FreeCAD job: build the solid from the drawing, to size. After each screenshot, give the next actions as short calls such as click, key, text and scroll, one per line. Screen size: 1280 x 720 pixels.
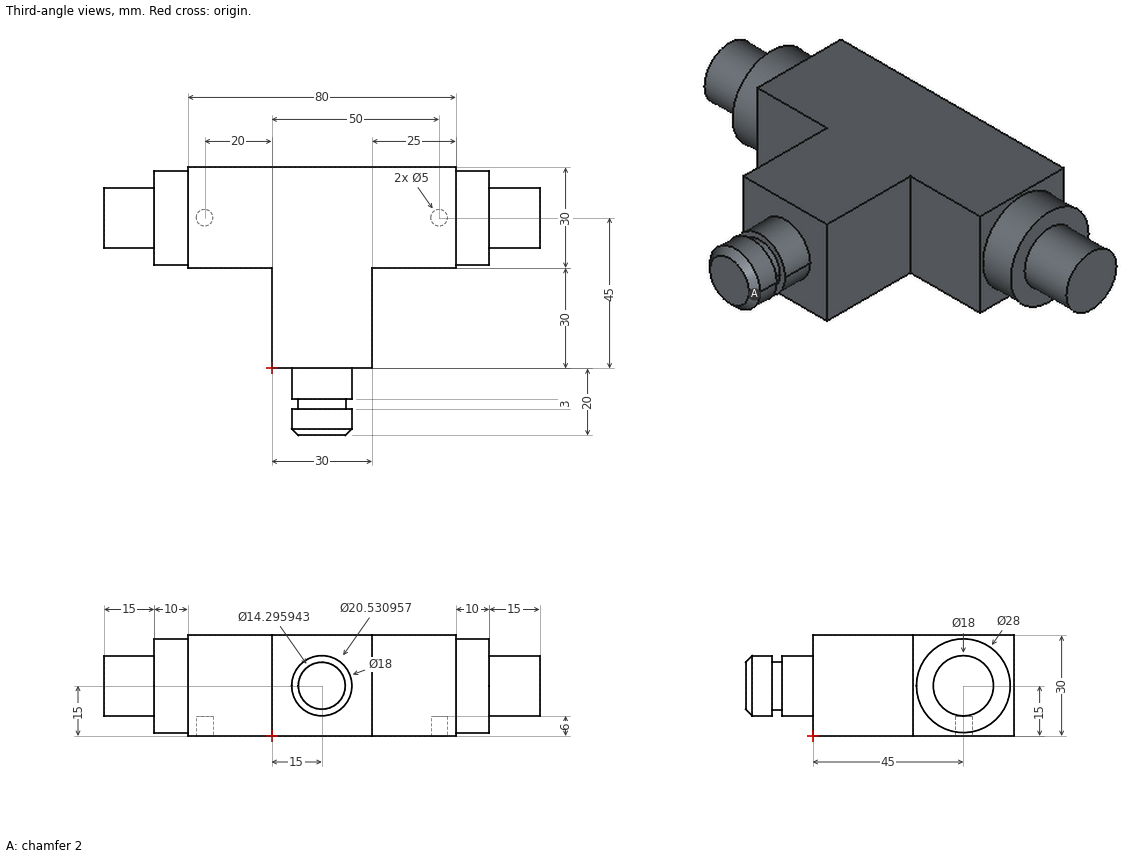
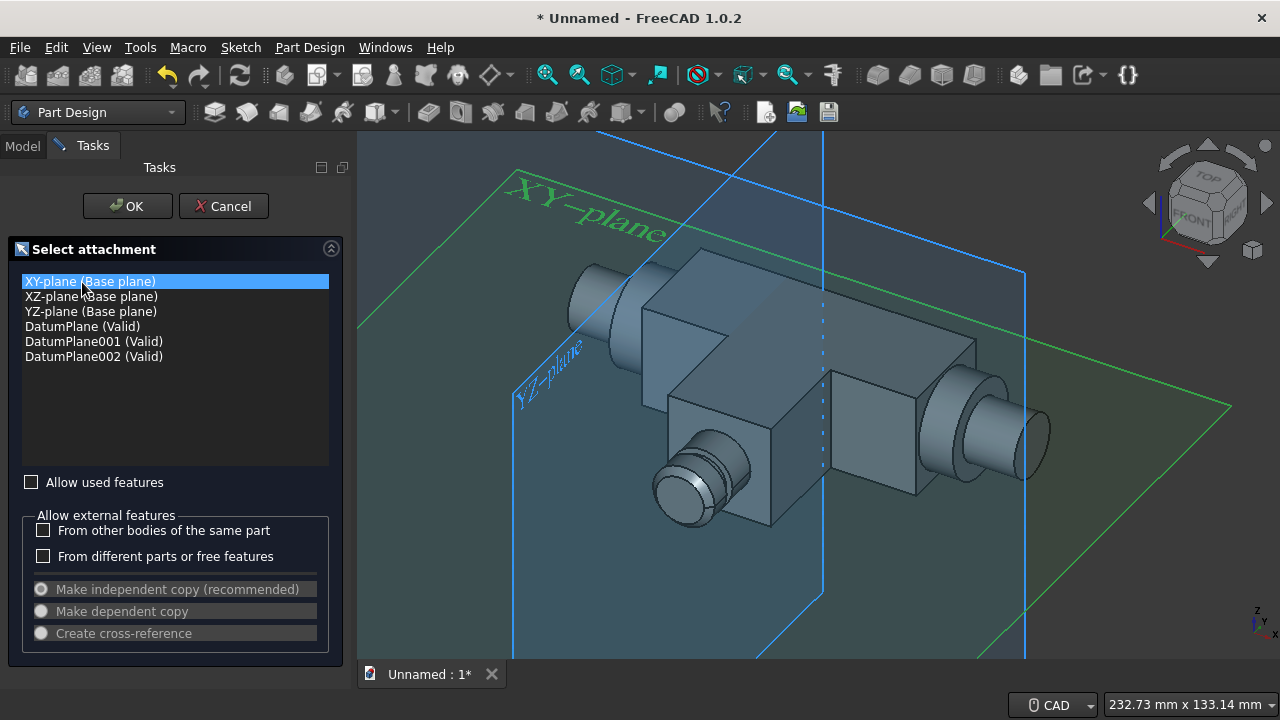
click(128, 206)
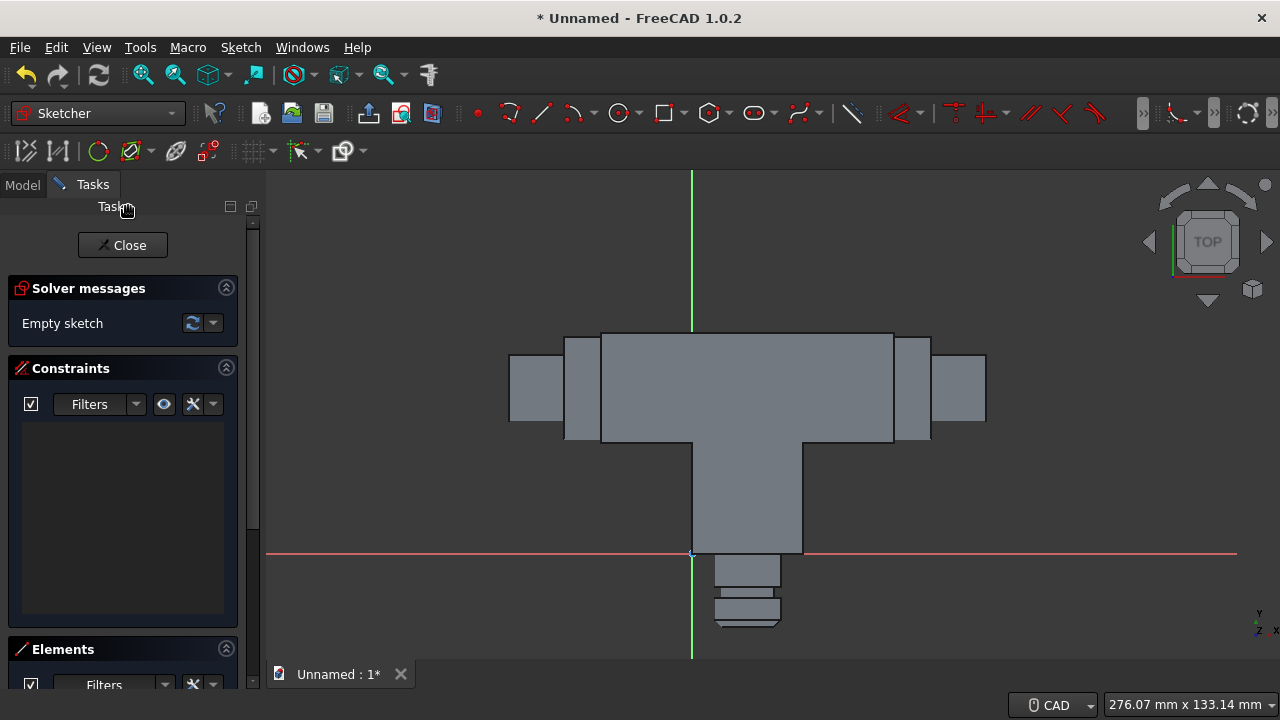
click(434, 114)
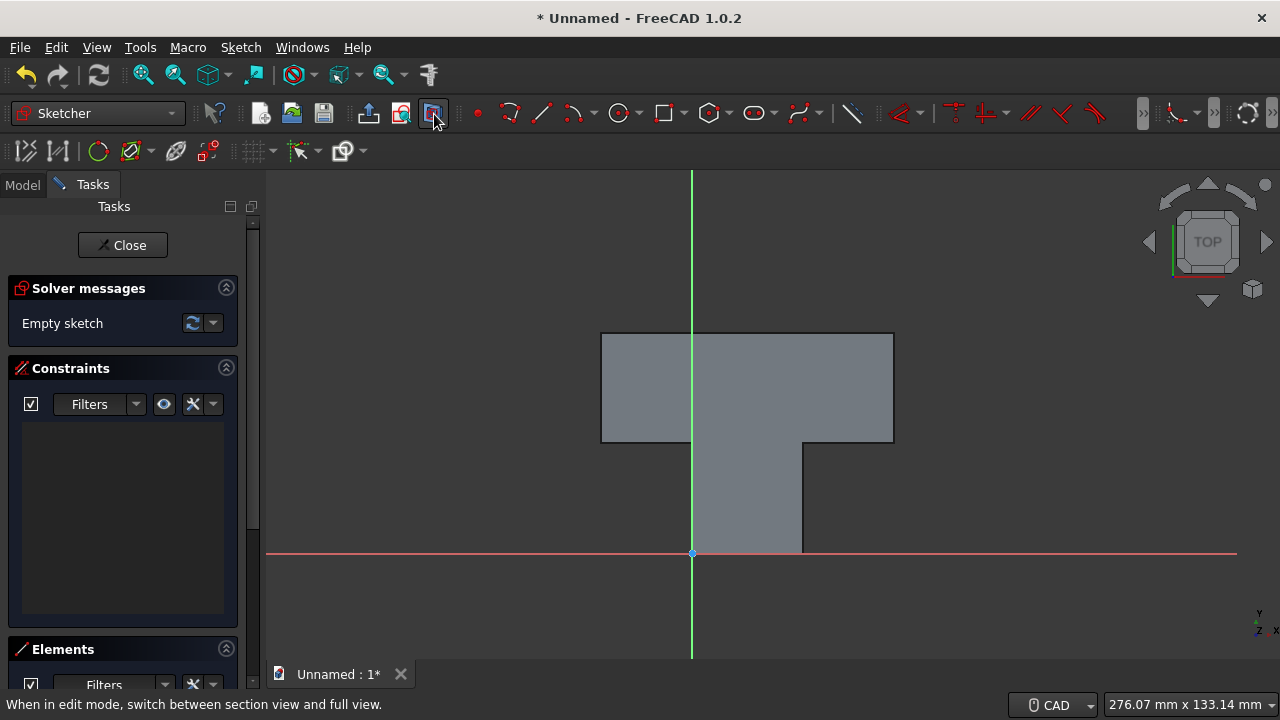
scroll(800, 530, up, 3)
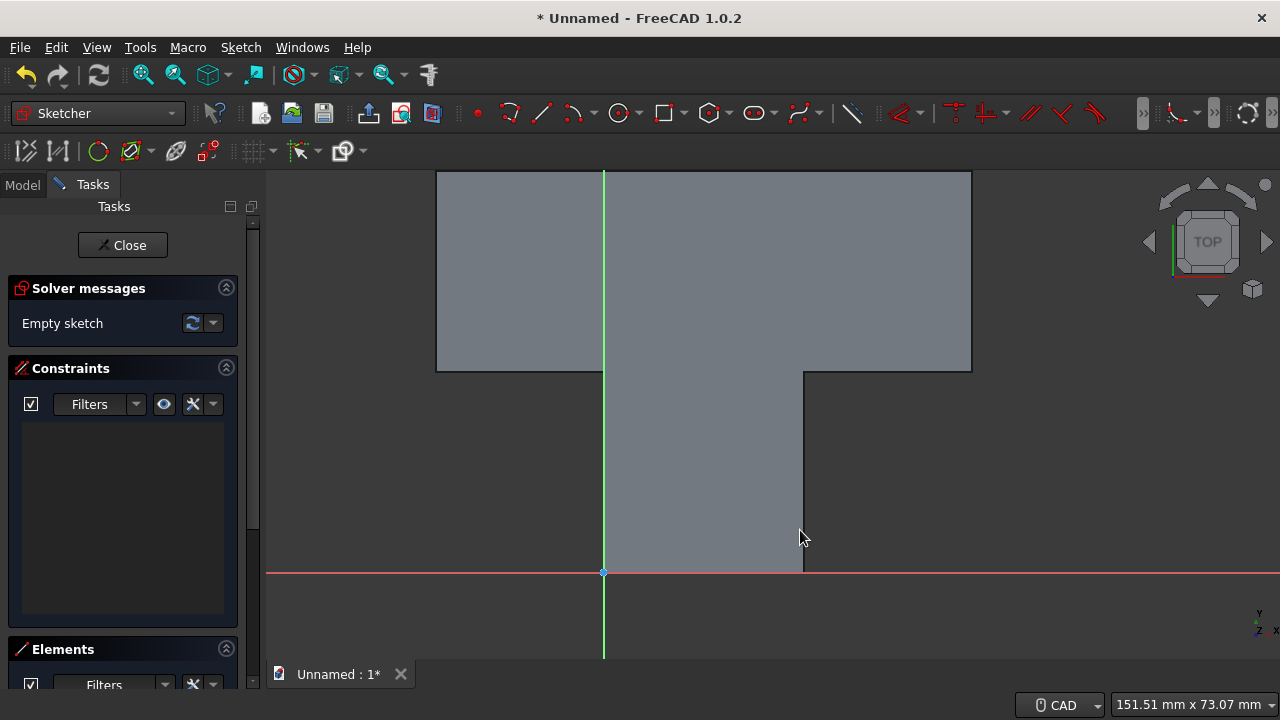
key(g)
key(c)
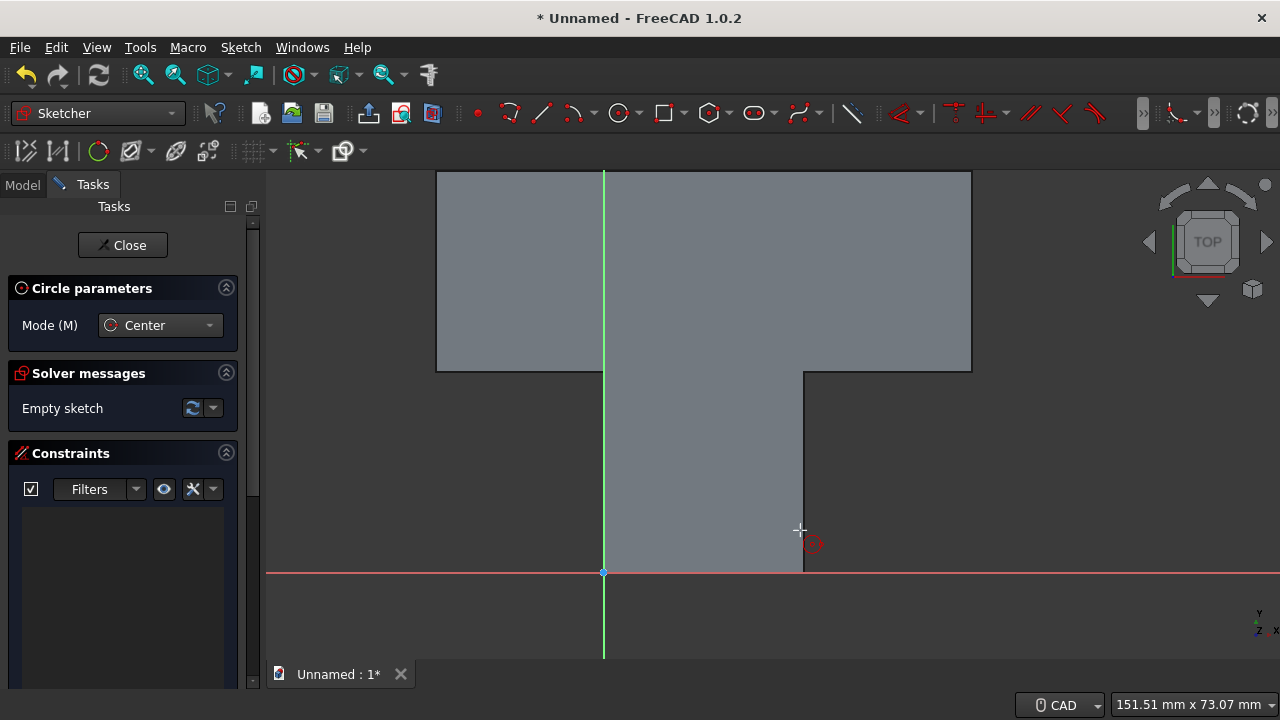
scroll(938, 271, up, 2)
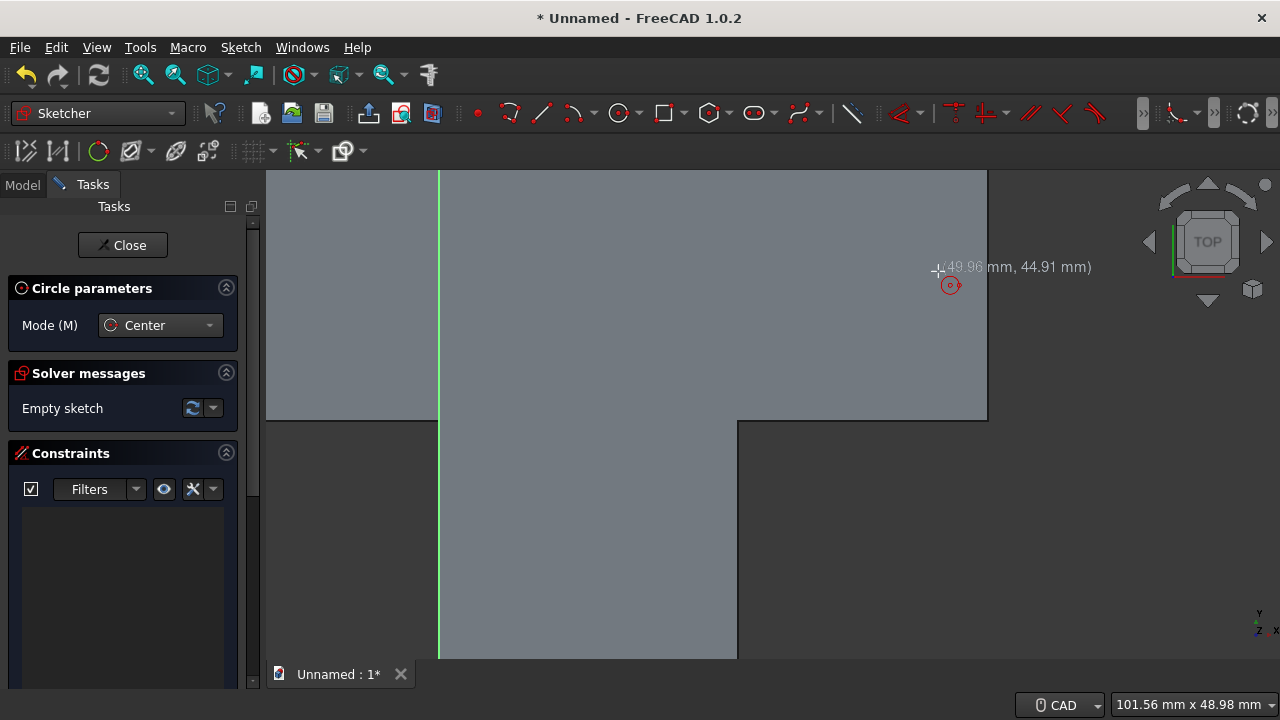
click(938, 271)
move(956, 254)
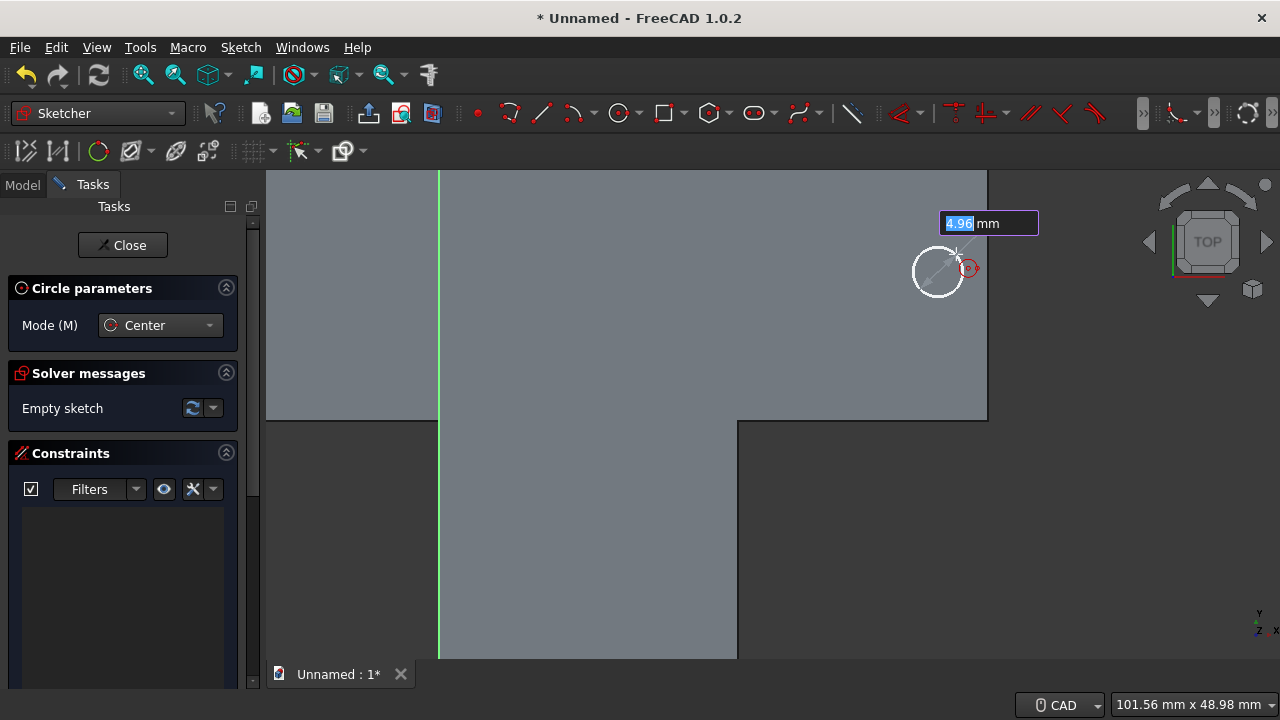
text(5)
key(Return)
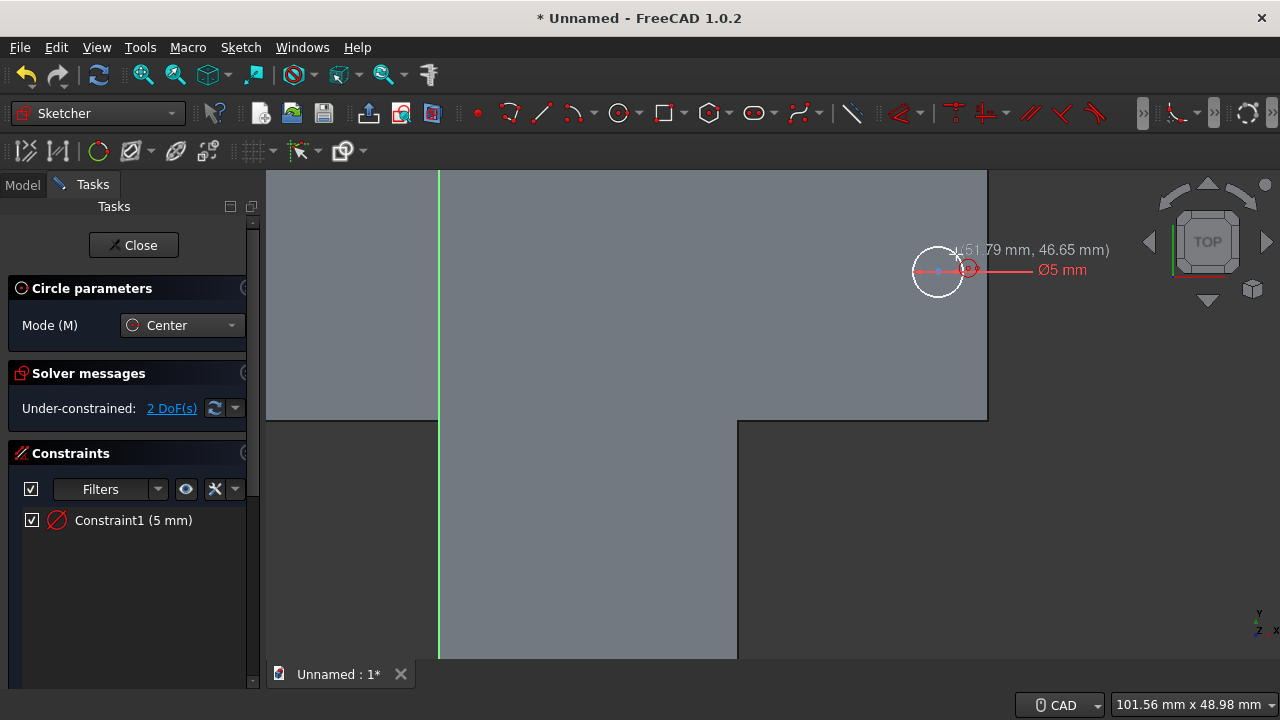
scroll(940, 274, down, 2)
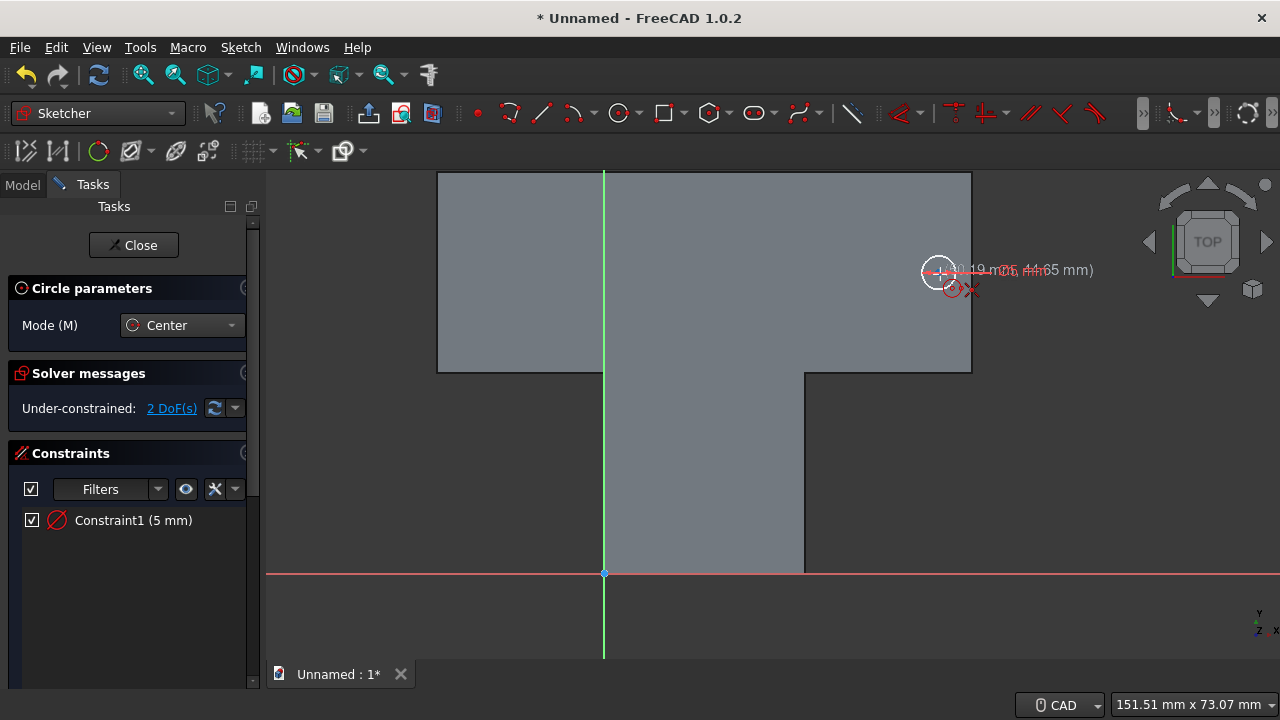
scroll(470, 272, up, 2)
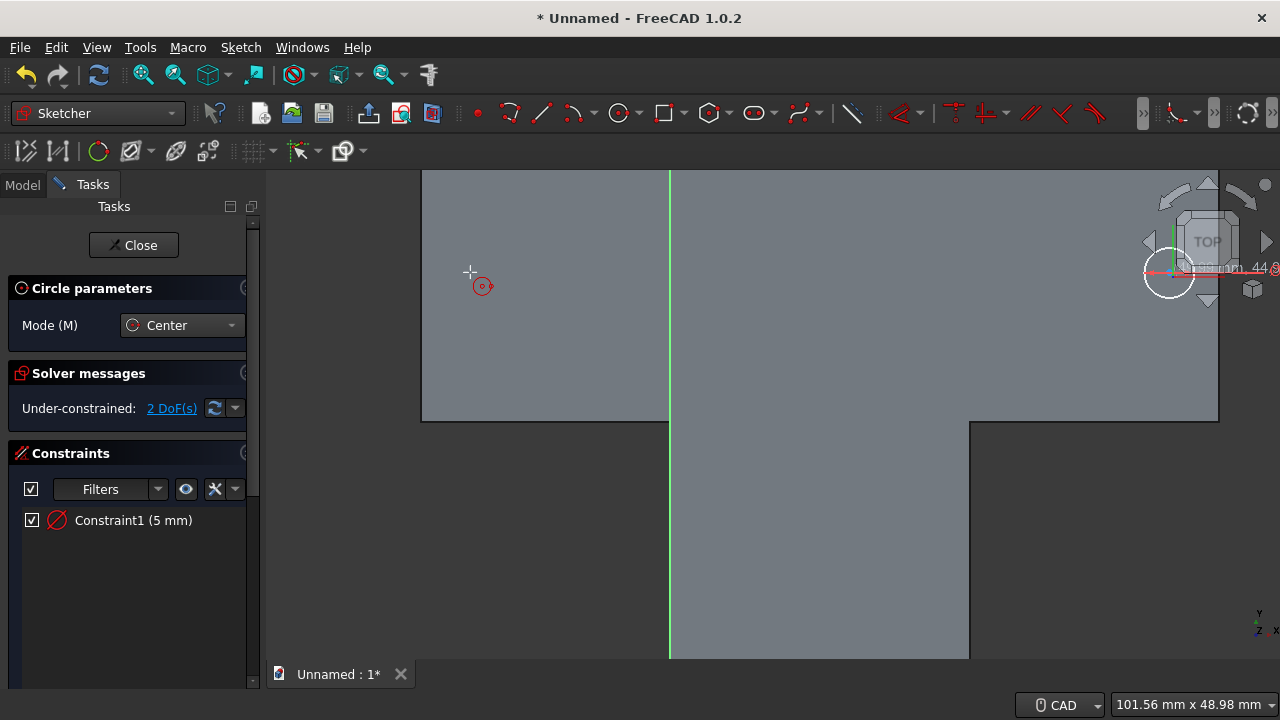
click(471, 272)
move(488, 255)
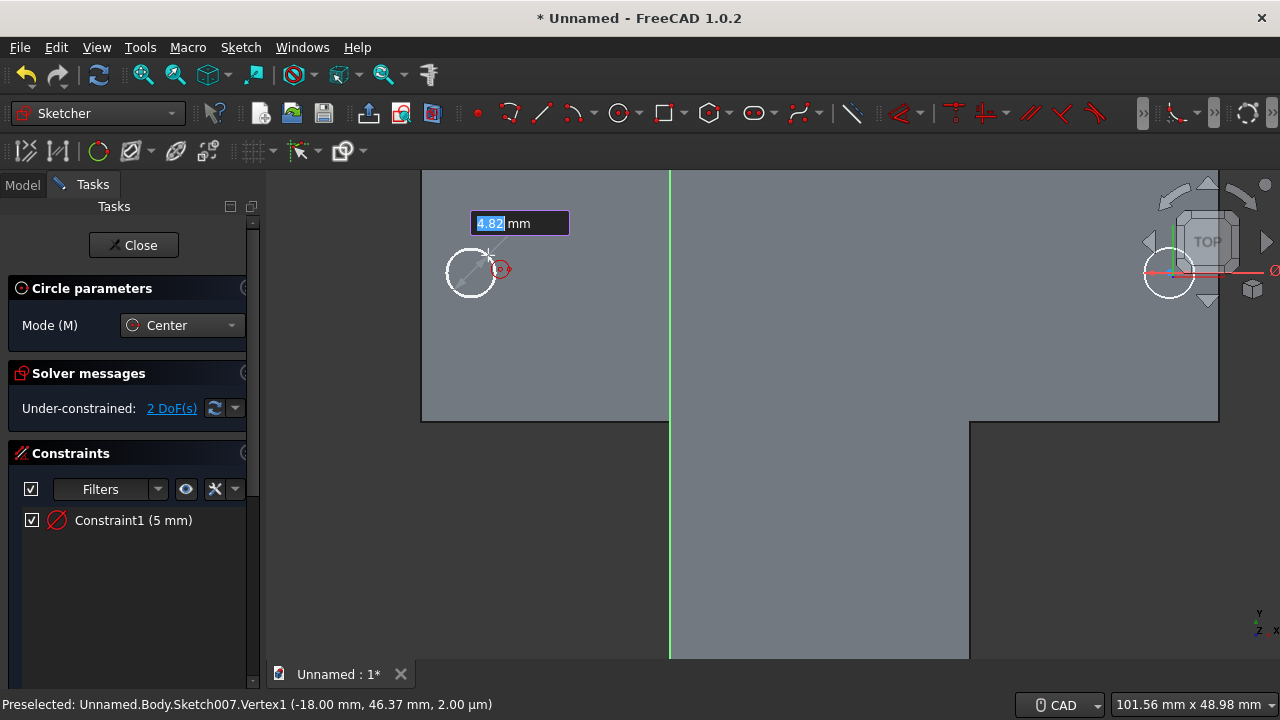
text(5)
key(Return)
key(Escape)